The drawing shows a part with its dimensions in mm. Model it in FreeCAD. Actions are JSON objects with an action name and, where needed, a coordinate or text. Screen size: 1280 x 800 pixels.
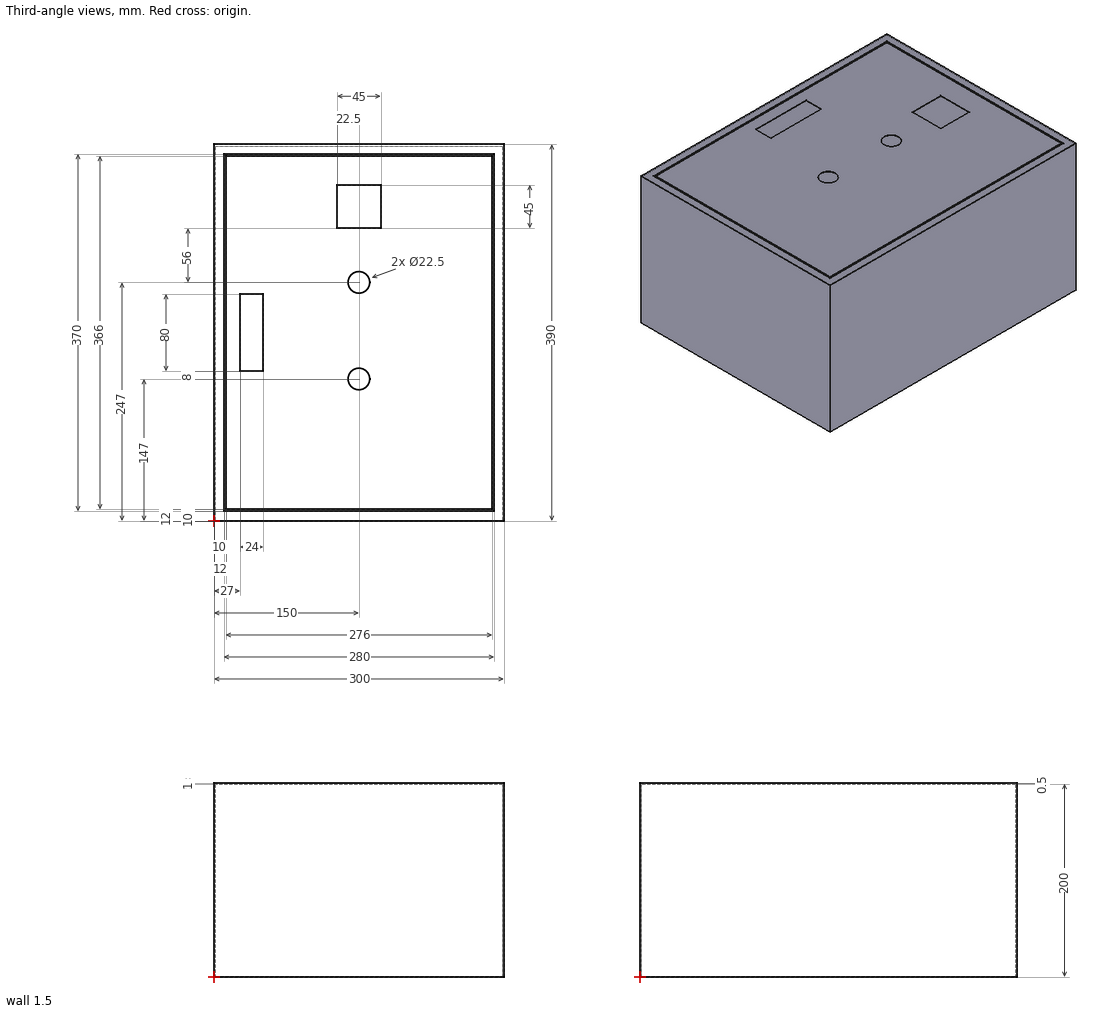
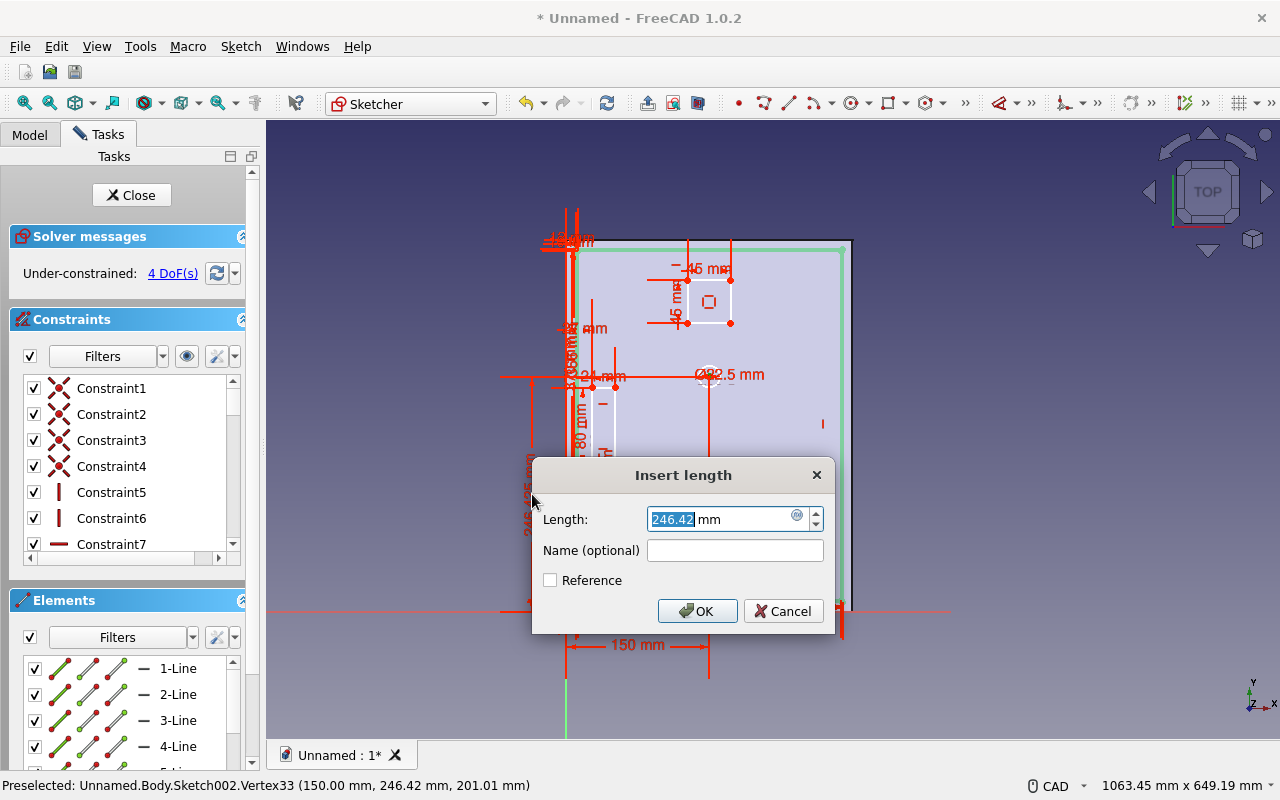
{"action": "type", "text": "247"}
{"action": "key", "text": "Return"}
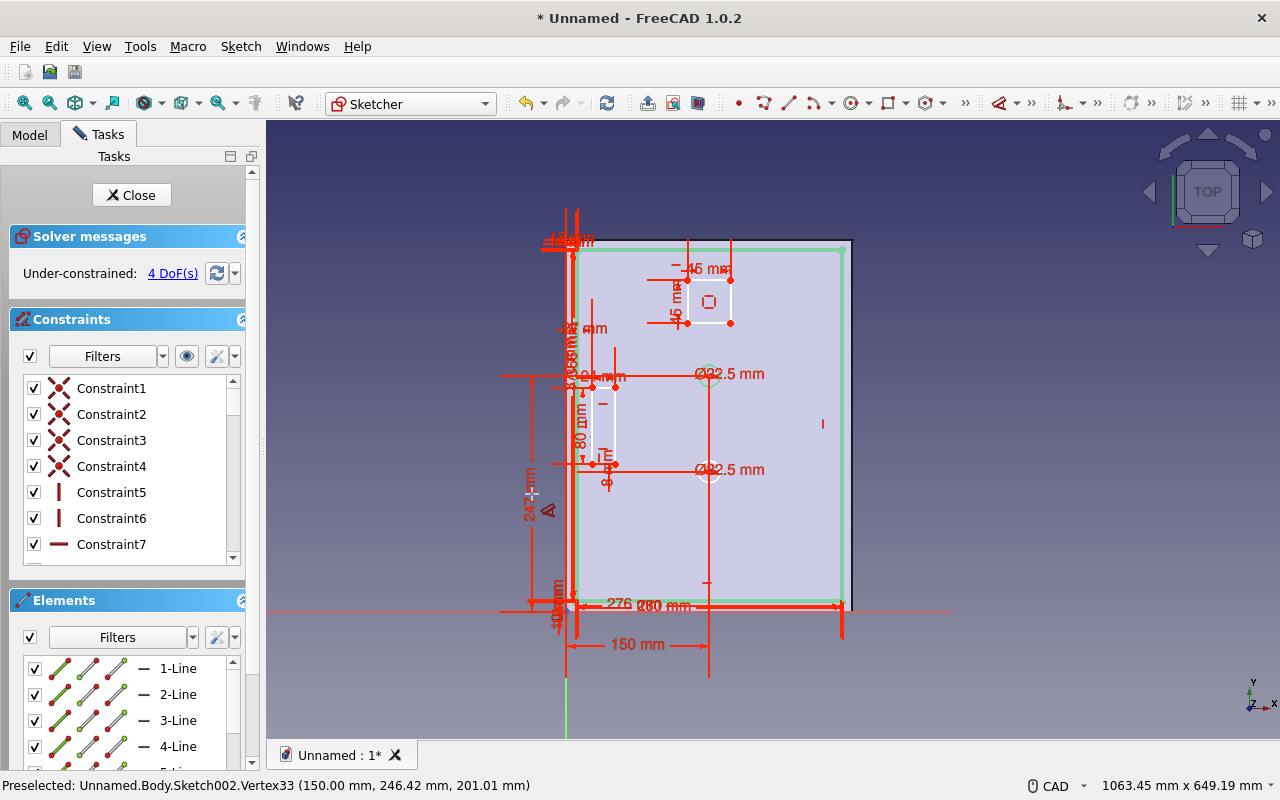
{"action": "left_click", "coordinate": [710, 472]}
{"action": "left_click", "coordinate": [638, 438]}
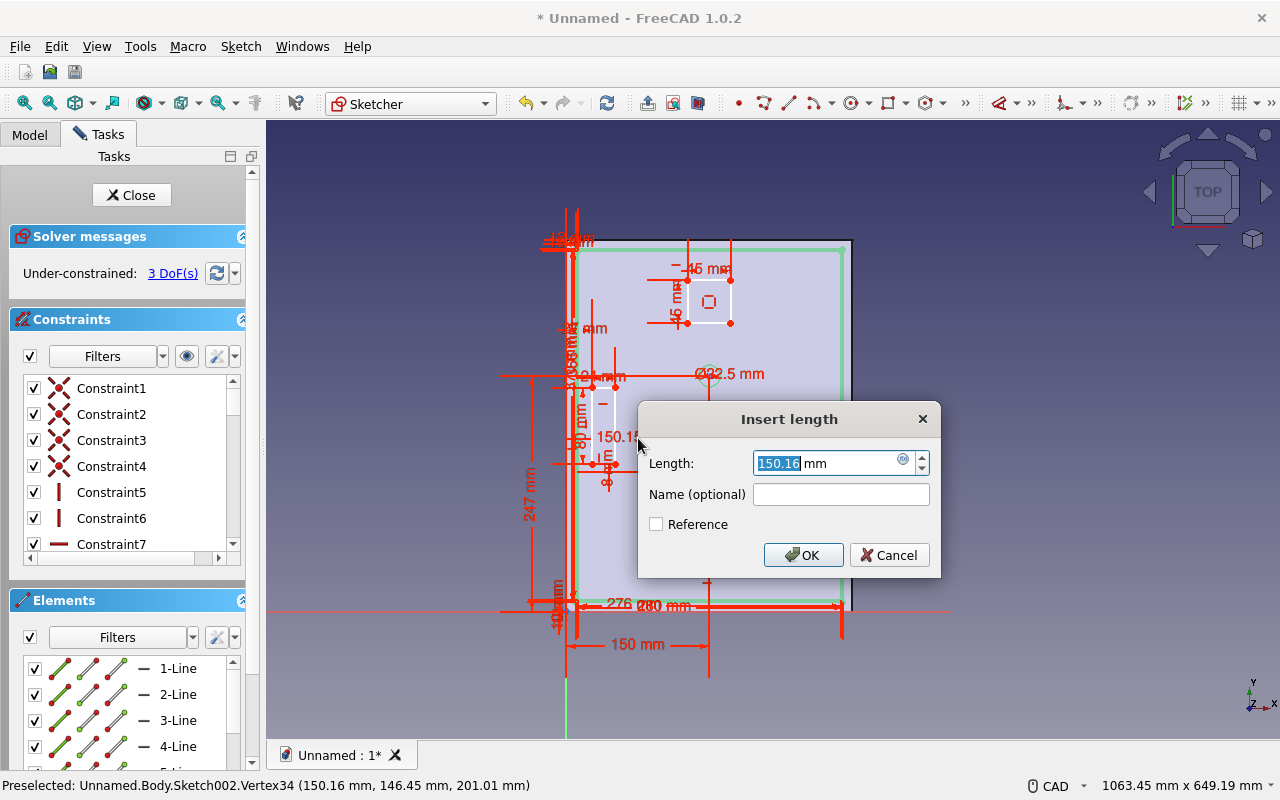
{"action": "type", "text": "150"}
{"action": "key", "text": "Return"}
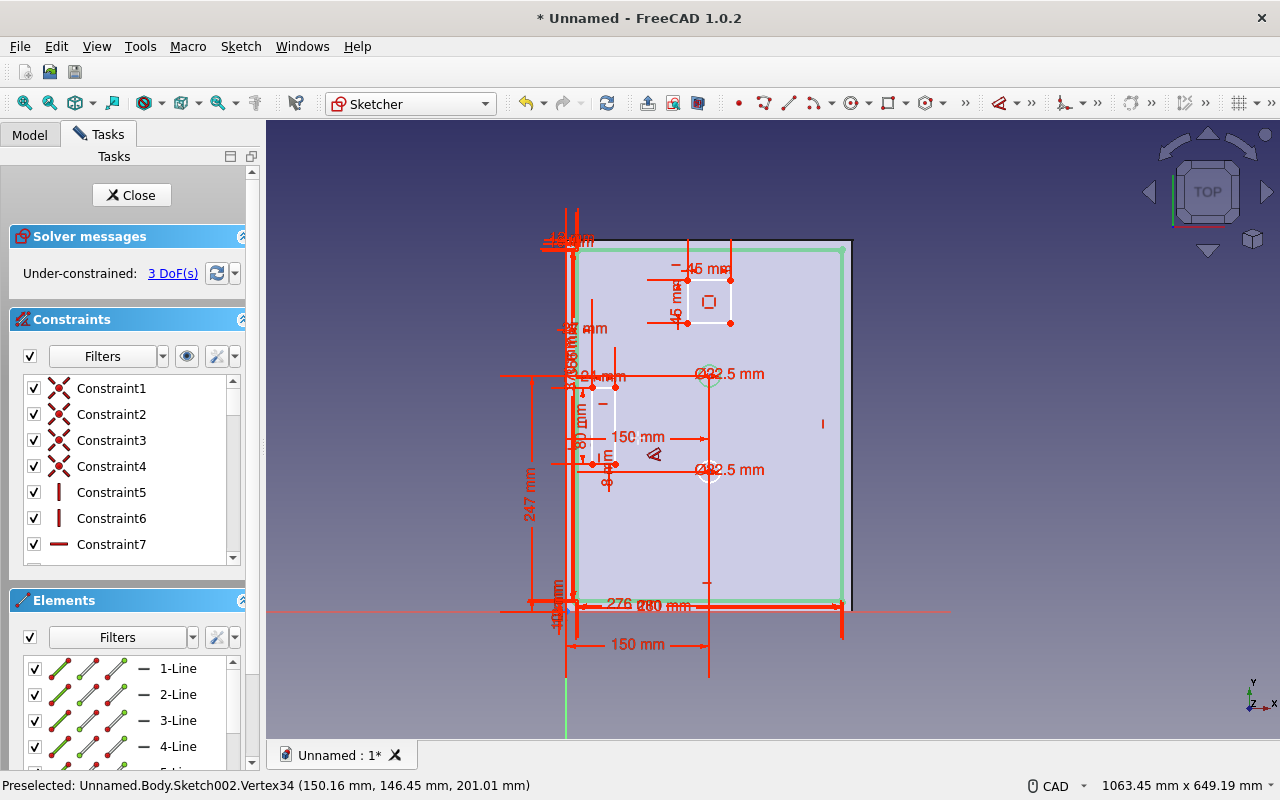
{"action": "left_click", "coordinate": [709, 472]}
{"action": "left_click", "coordinate": [532, 542]}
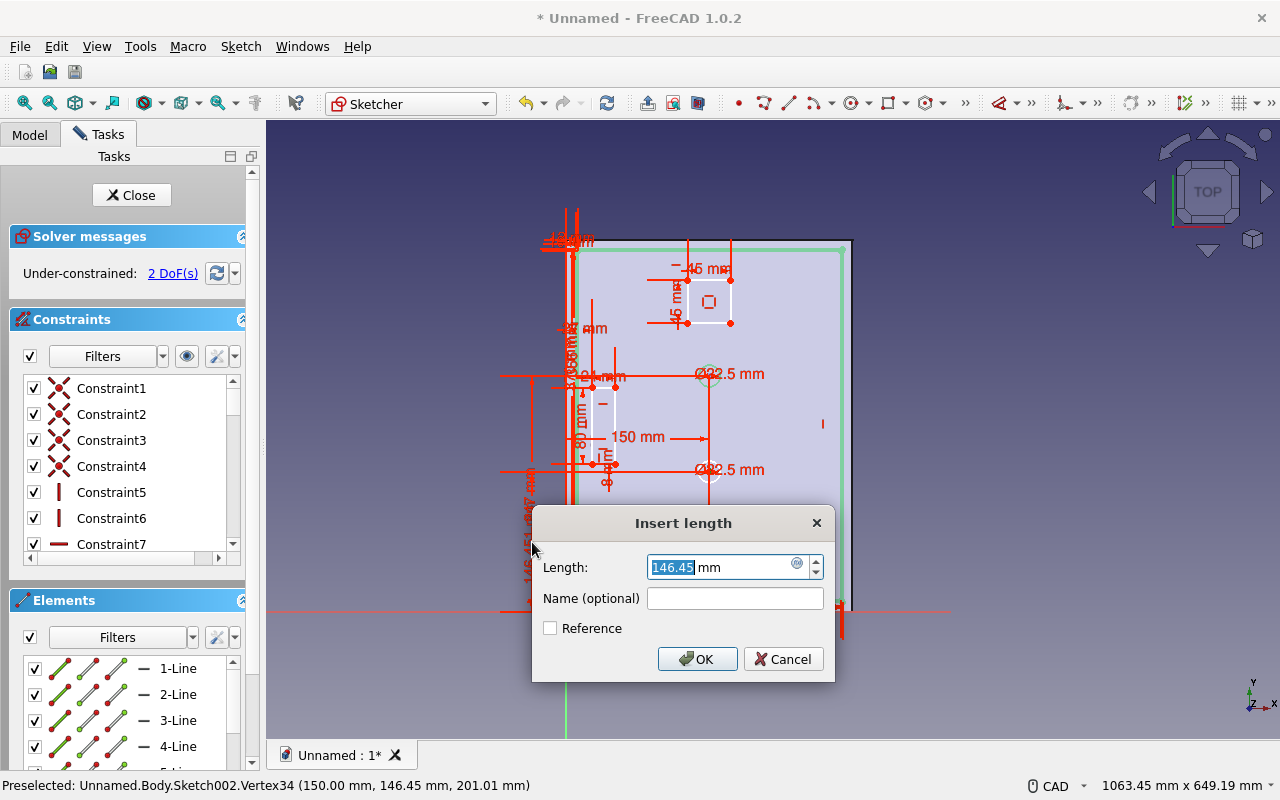
{"action": "type", "text": "147"}
{"action": "key", "text": "Return"}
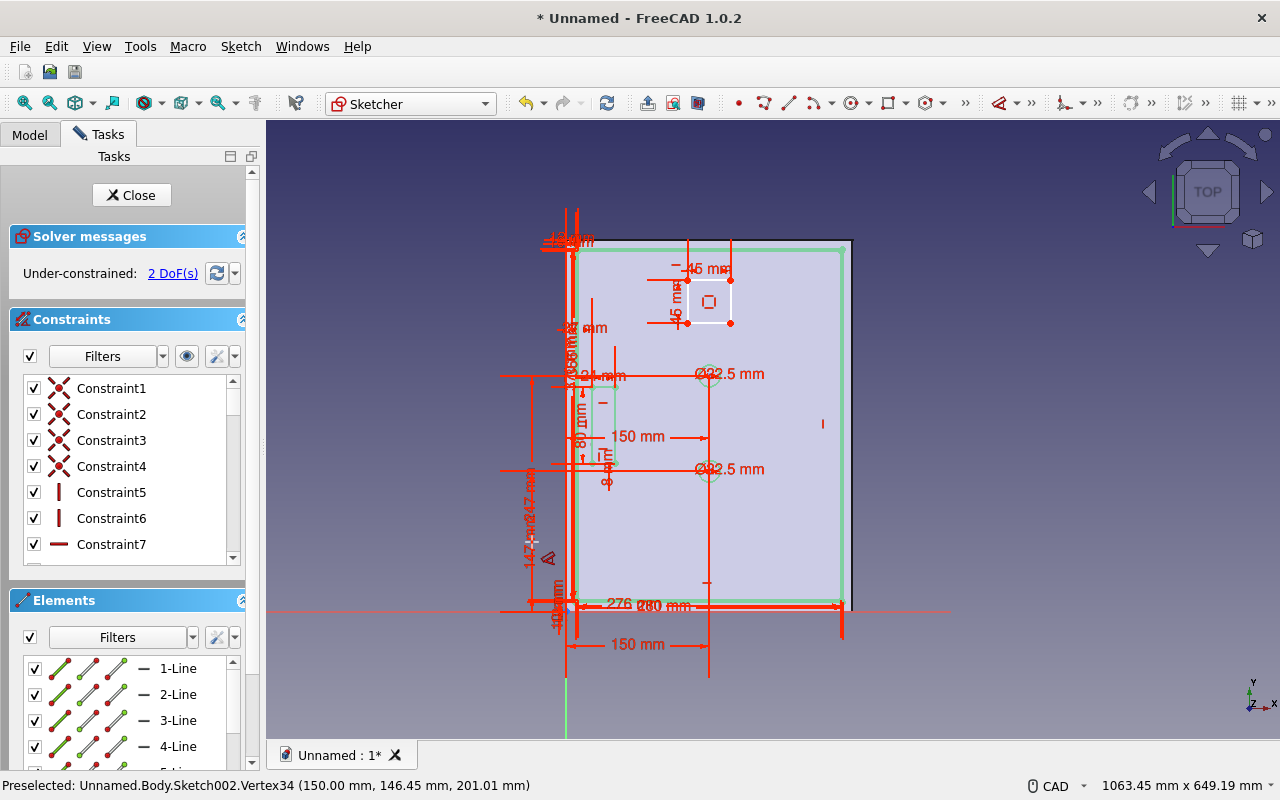
{"action": "left_click", "coordinate": [688, 323]}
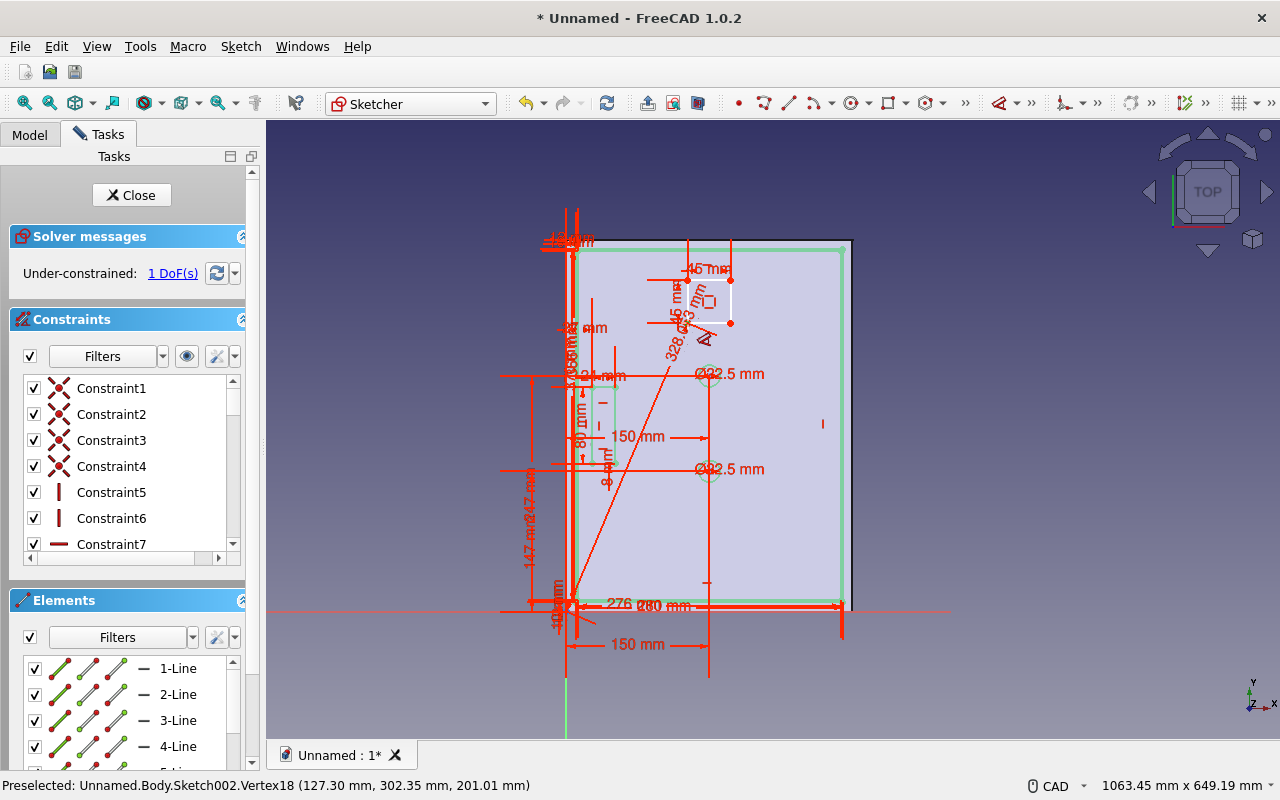
{"action": "left_click", "coordinate": [709, 376]}
{"action": "left_click", "coordinate": [654, 362]}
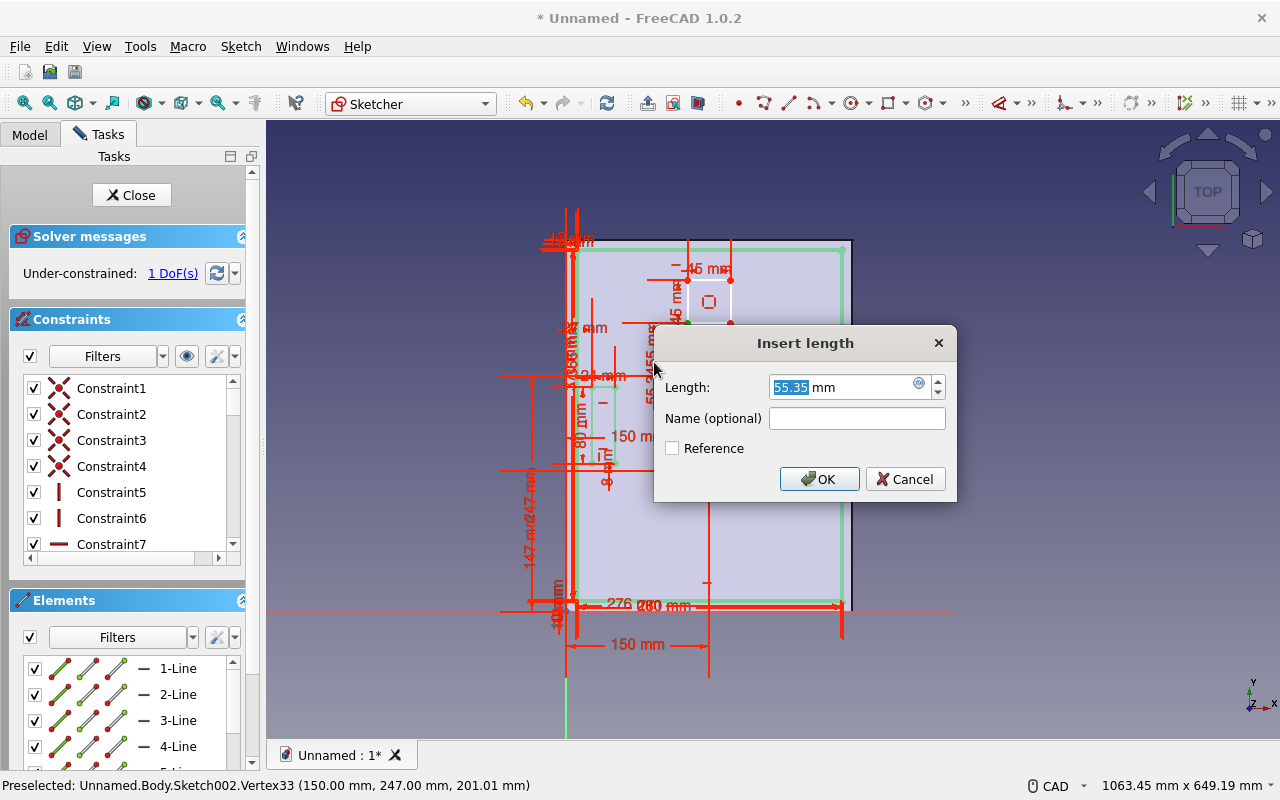
{"action": "type", "text": "56"}
{"action": "key", "text": "Return"}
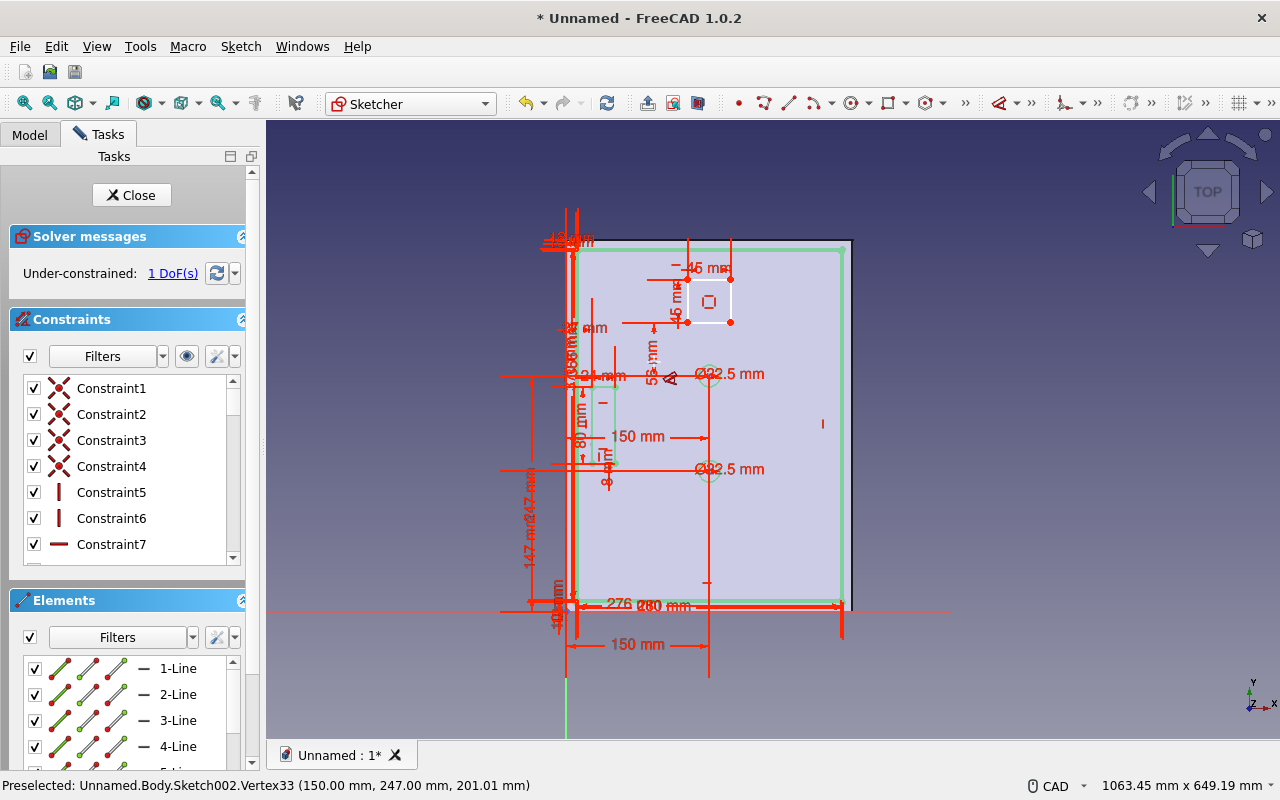
{"action": "scroll", "coordinate": [688, 323], "scroll_direction": "up", "scroll_amount": 4}